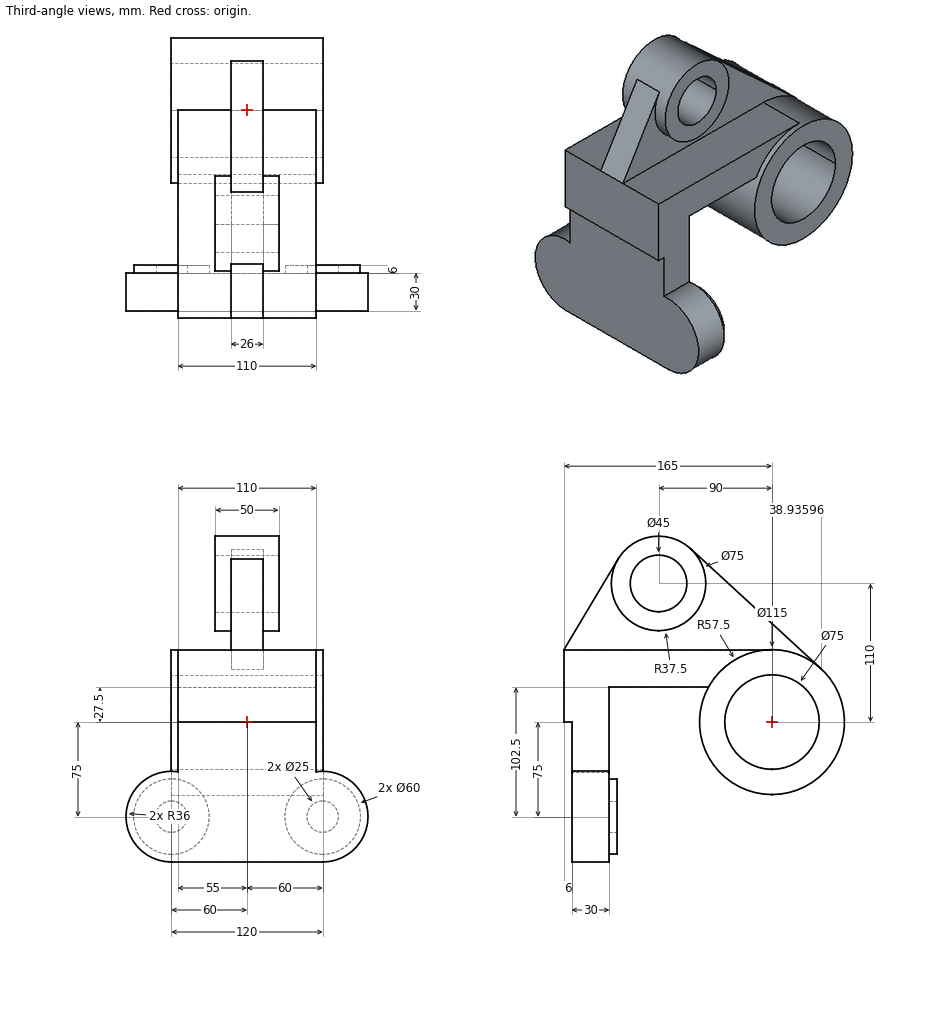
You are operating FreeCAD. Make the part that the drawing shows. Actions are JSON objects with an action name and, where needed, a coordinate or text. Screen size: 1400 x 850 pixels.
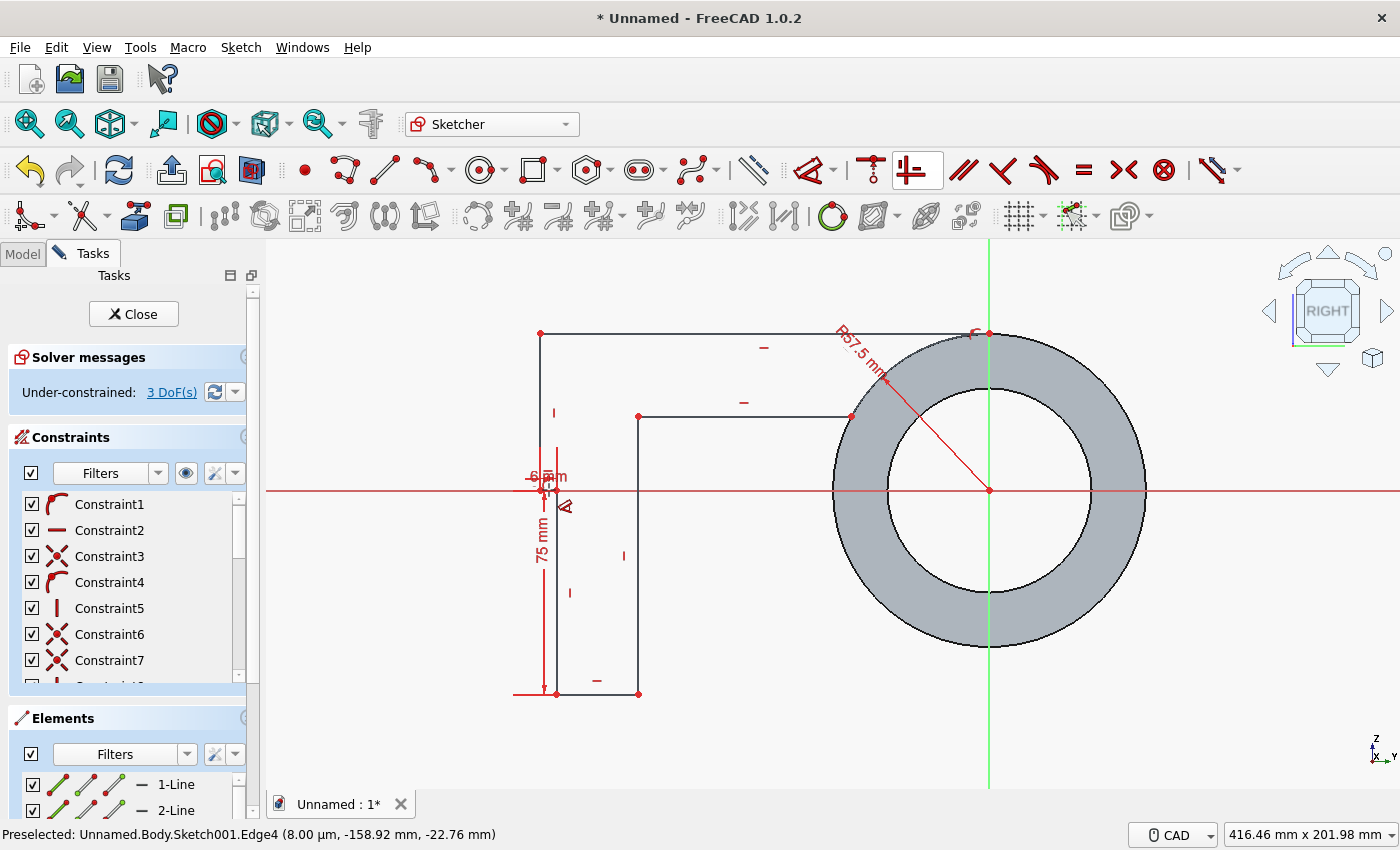
{"action": "left_click", "coordinate": [581, 695]}
{"action": "left_click", "coordinate": [598, 729]}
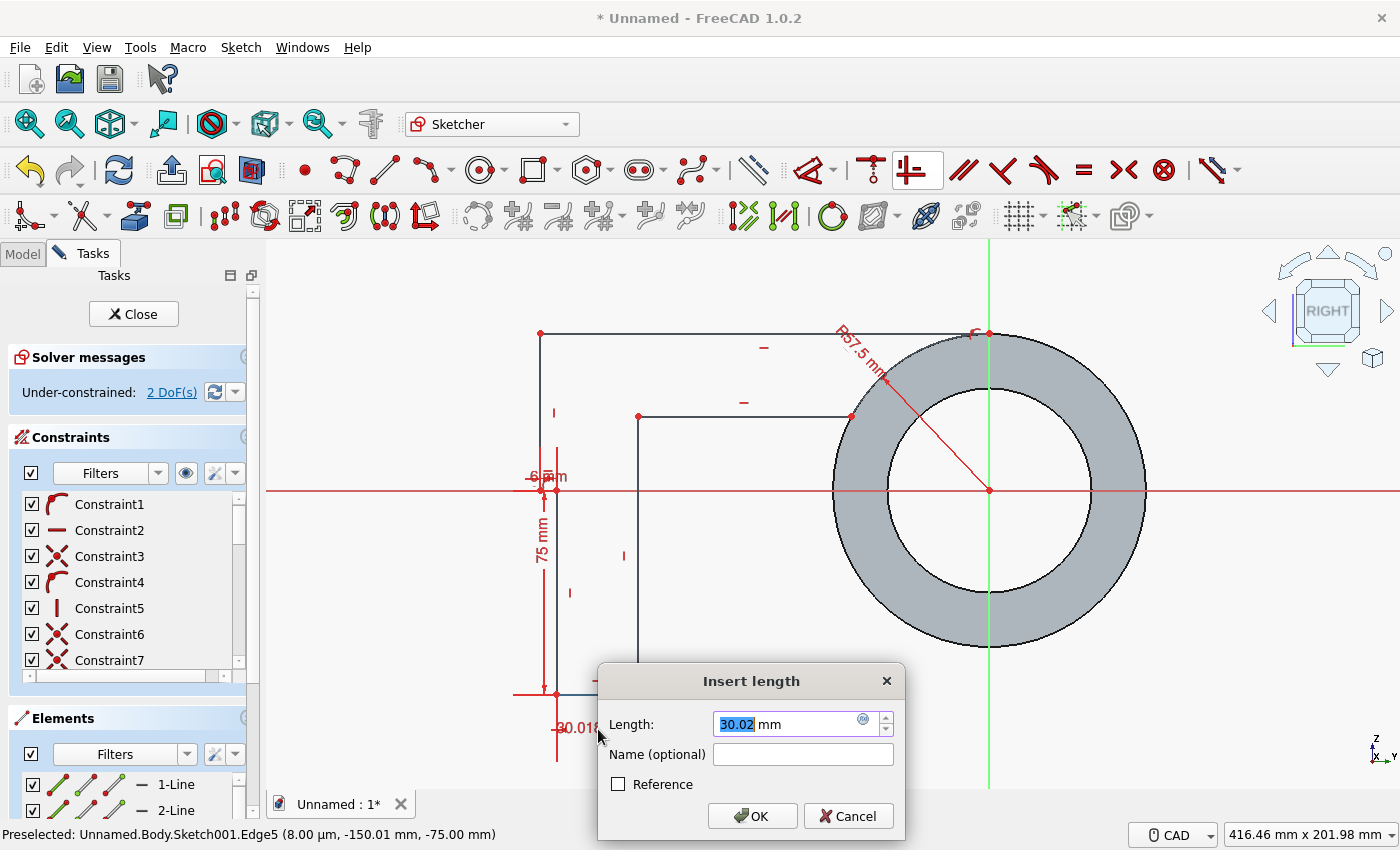
{"action": "type", "text": "30"}
{"action": "key", "text": "Return"}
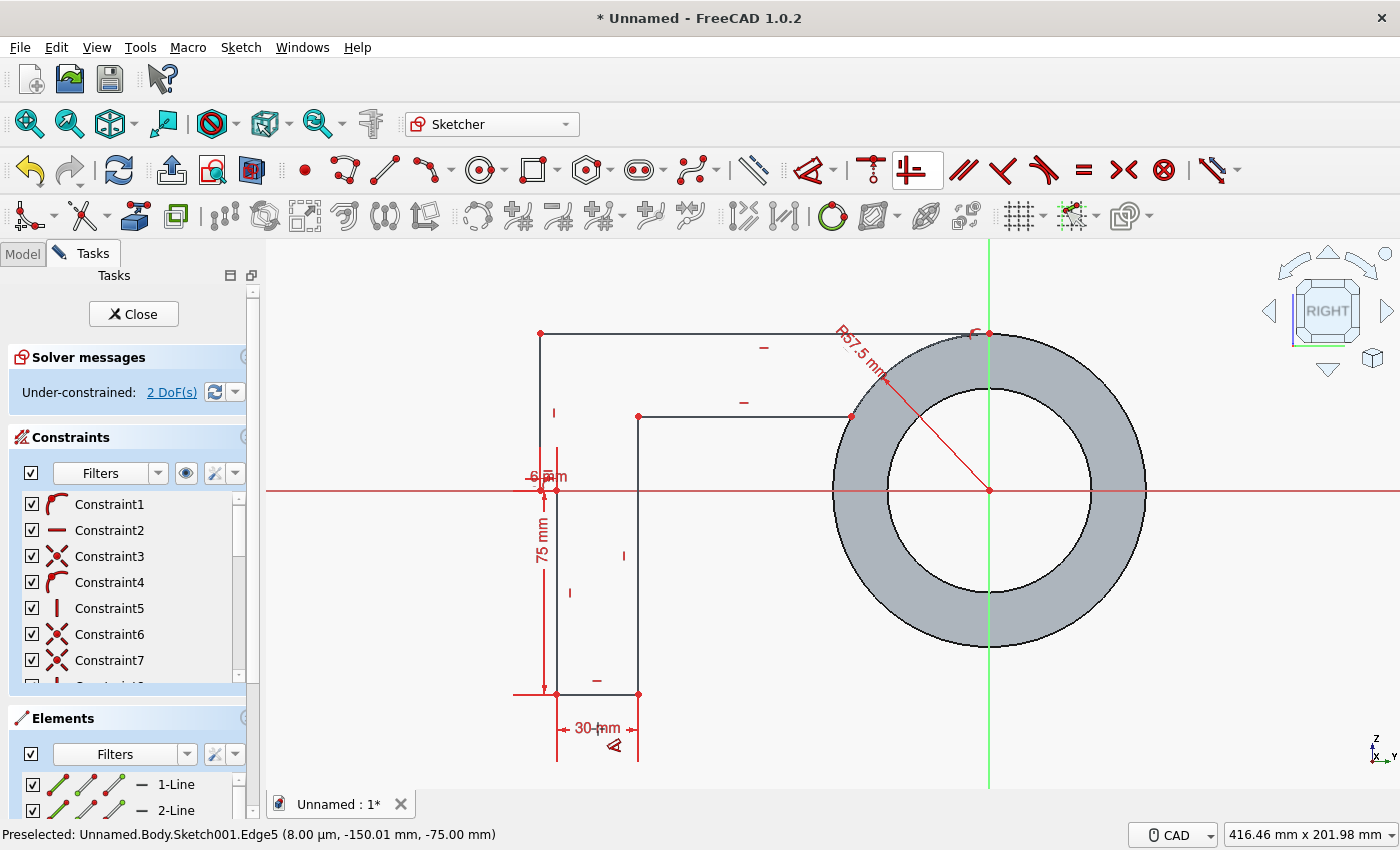
{"action": "left_click", "coordinate": [855, 334]}
{"action": "left_click", "coordinate": [765, 300]}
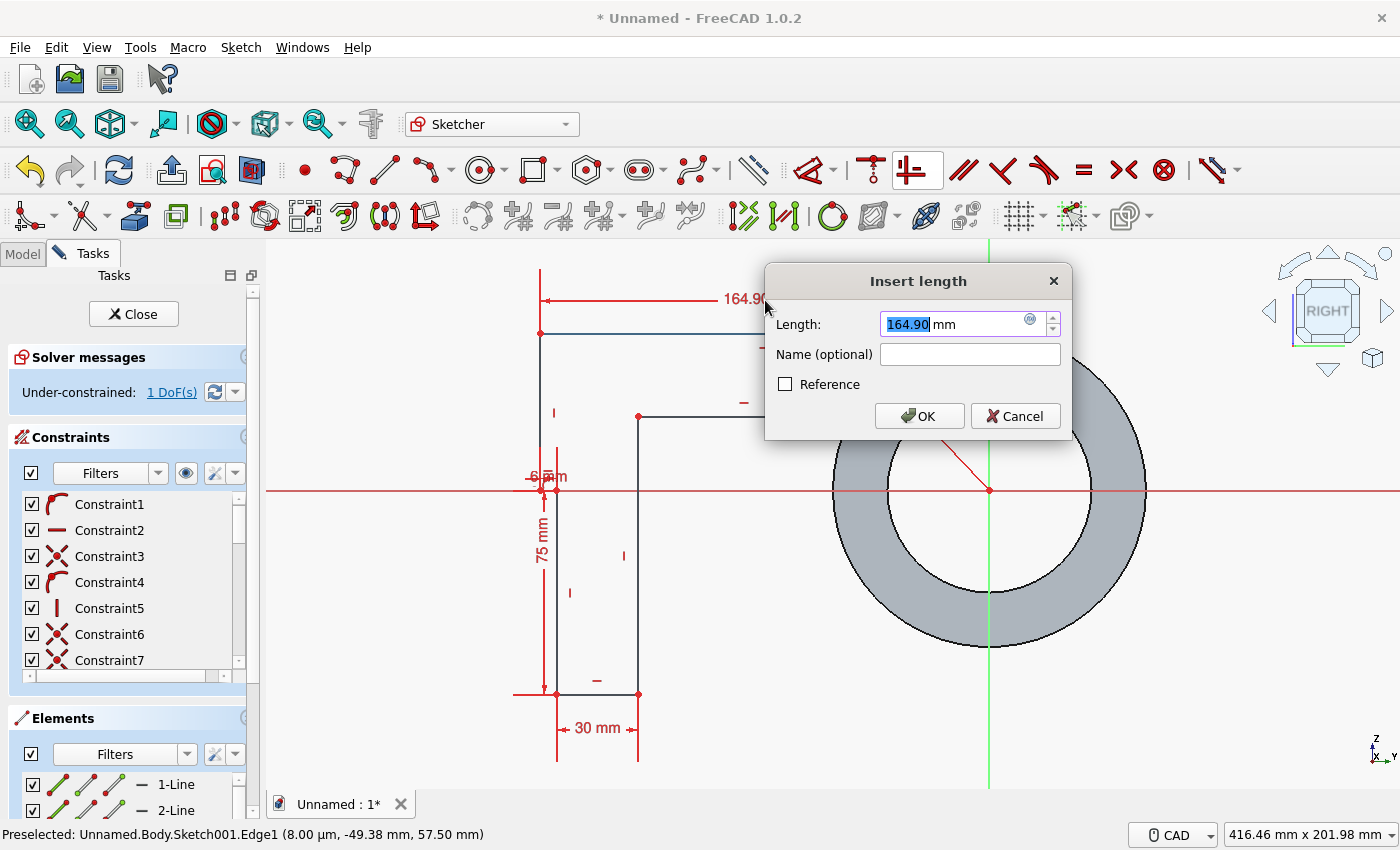
{"action": "type", "text": "165"}
{"action": "key", "text": "Return"}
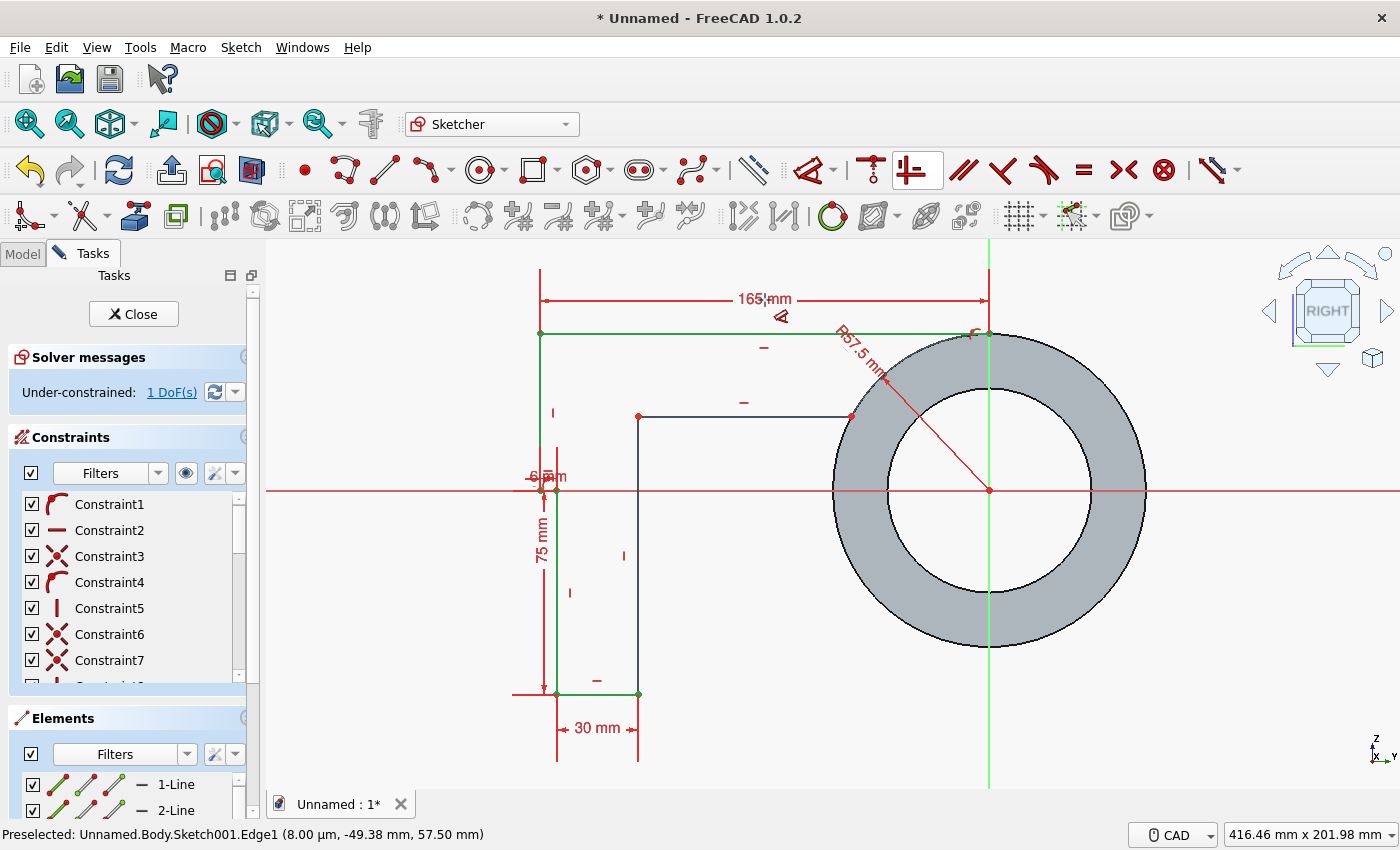
{"action": "left_click", "coordinate": [638, 611]}
{"action": "left_click", "coordinate": [604, 620]}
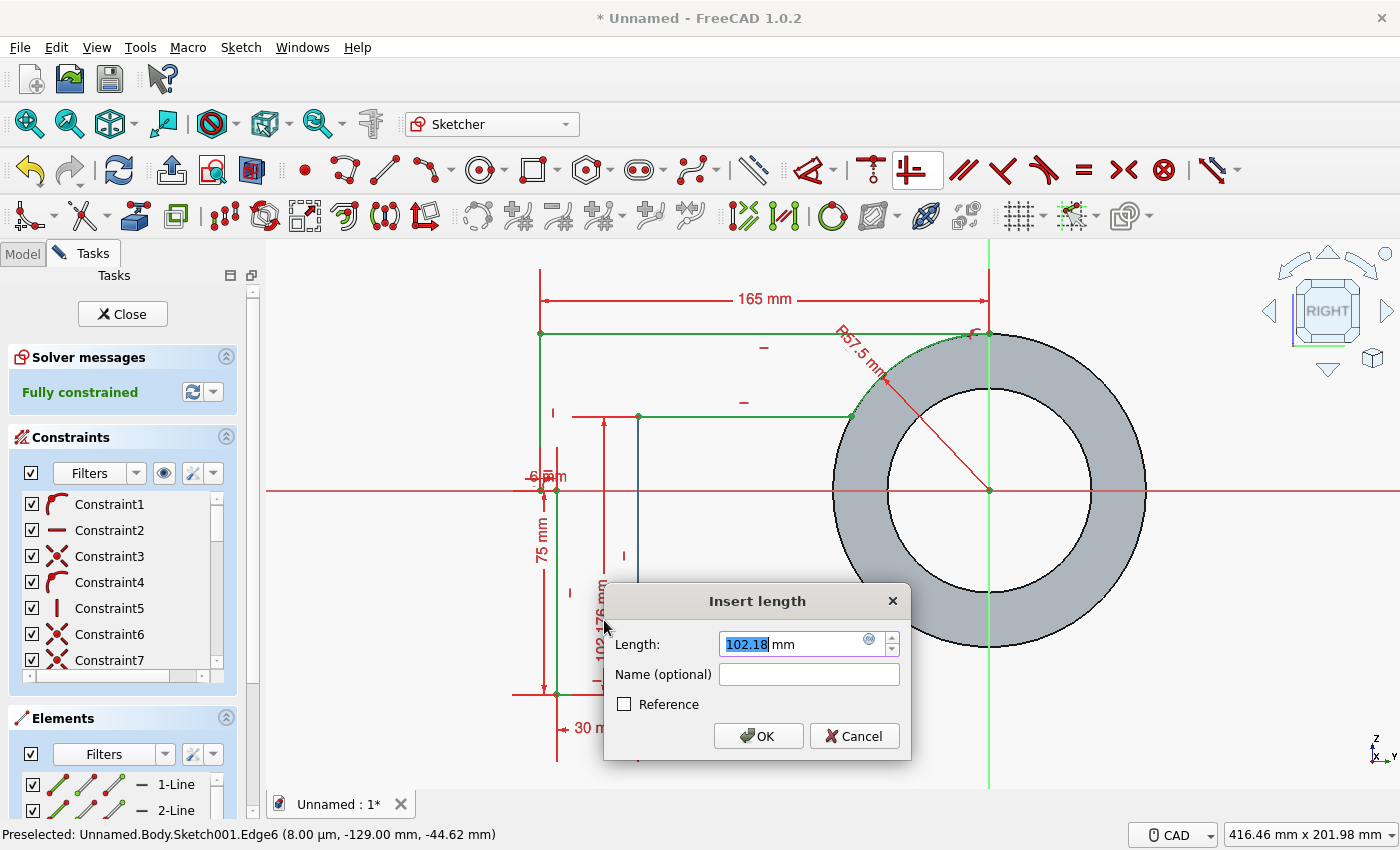
{"action": "type", "text": "102.5"}
{"action": "key", "text": "Return"}
{"action": "key", "text": "Escape"}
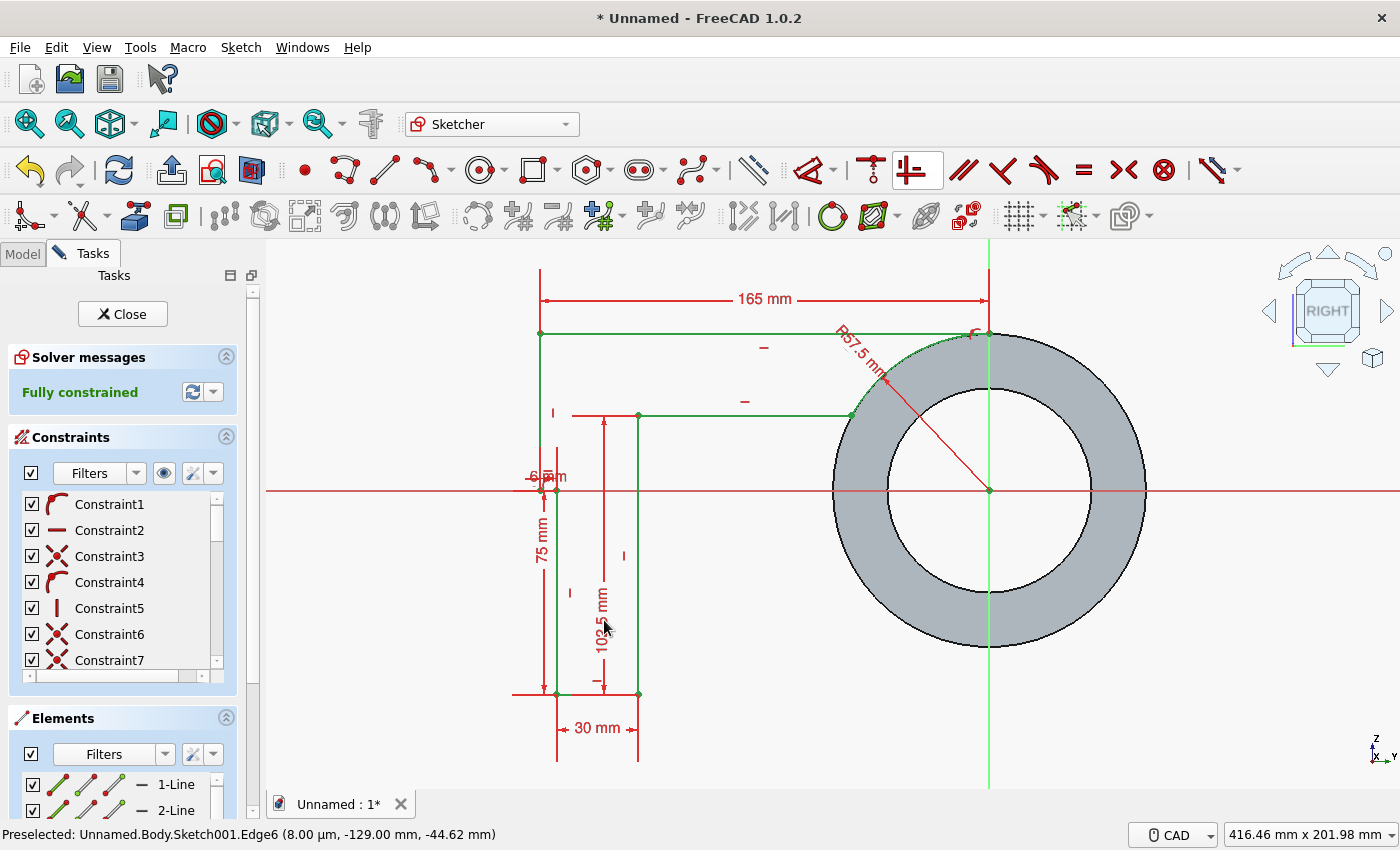
{"action": "left_click", "coordinate": [123, 314]}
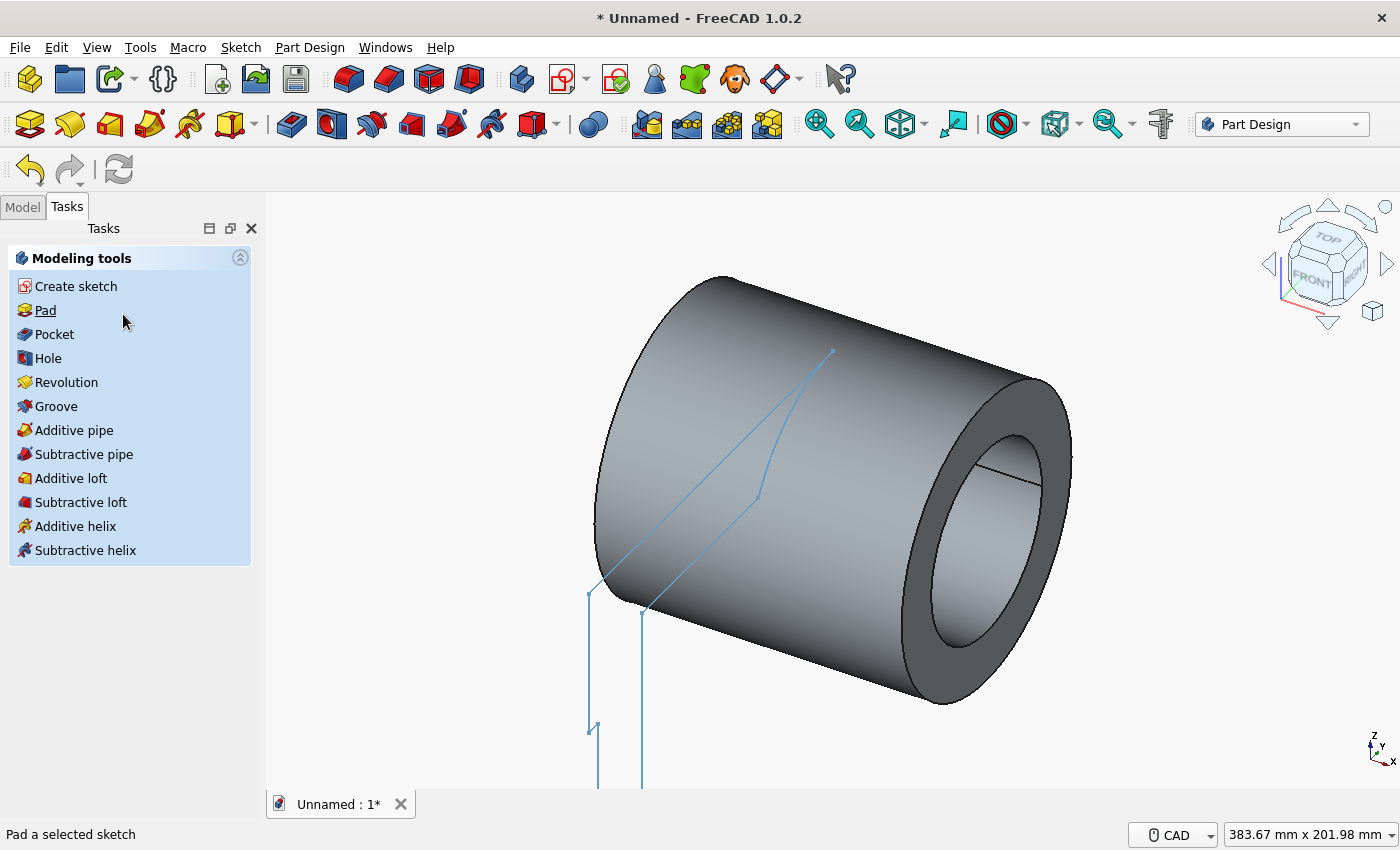
{"action": "left_click", "coordinate": [30, 124]}